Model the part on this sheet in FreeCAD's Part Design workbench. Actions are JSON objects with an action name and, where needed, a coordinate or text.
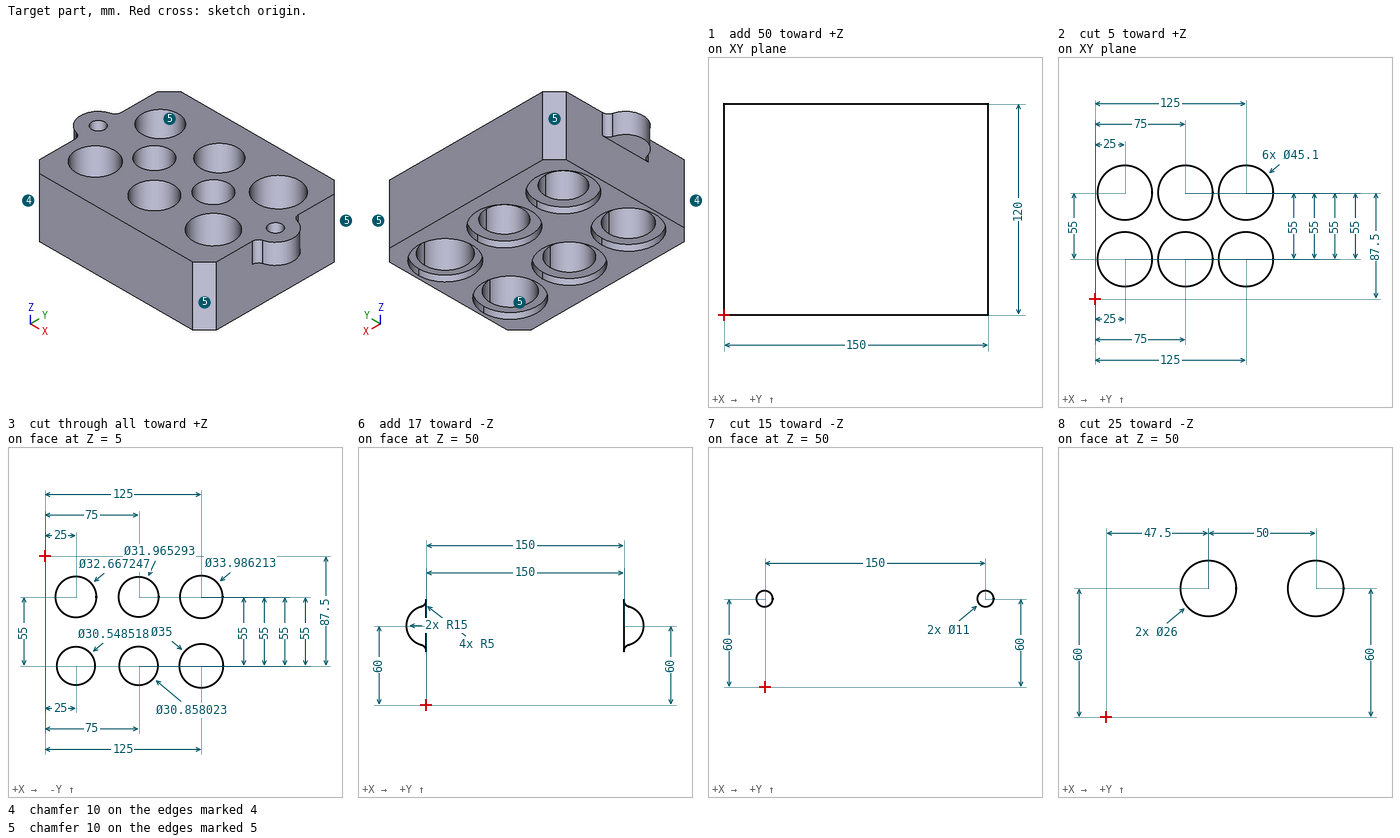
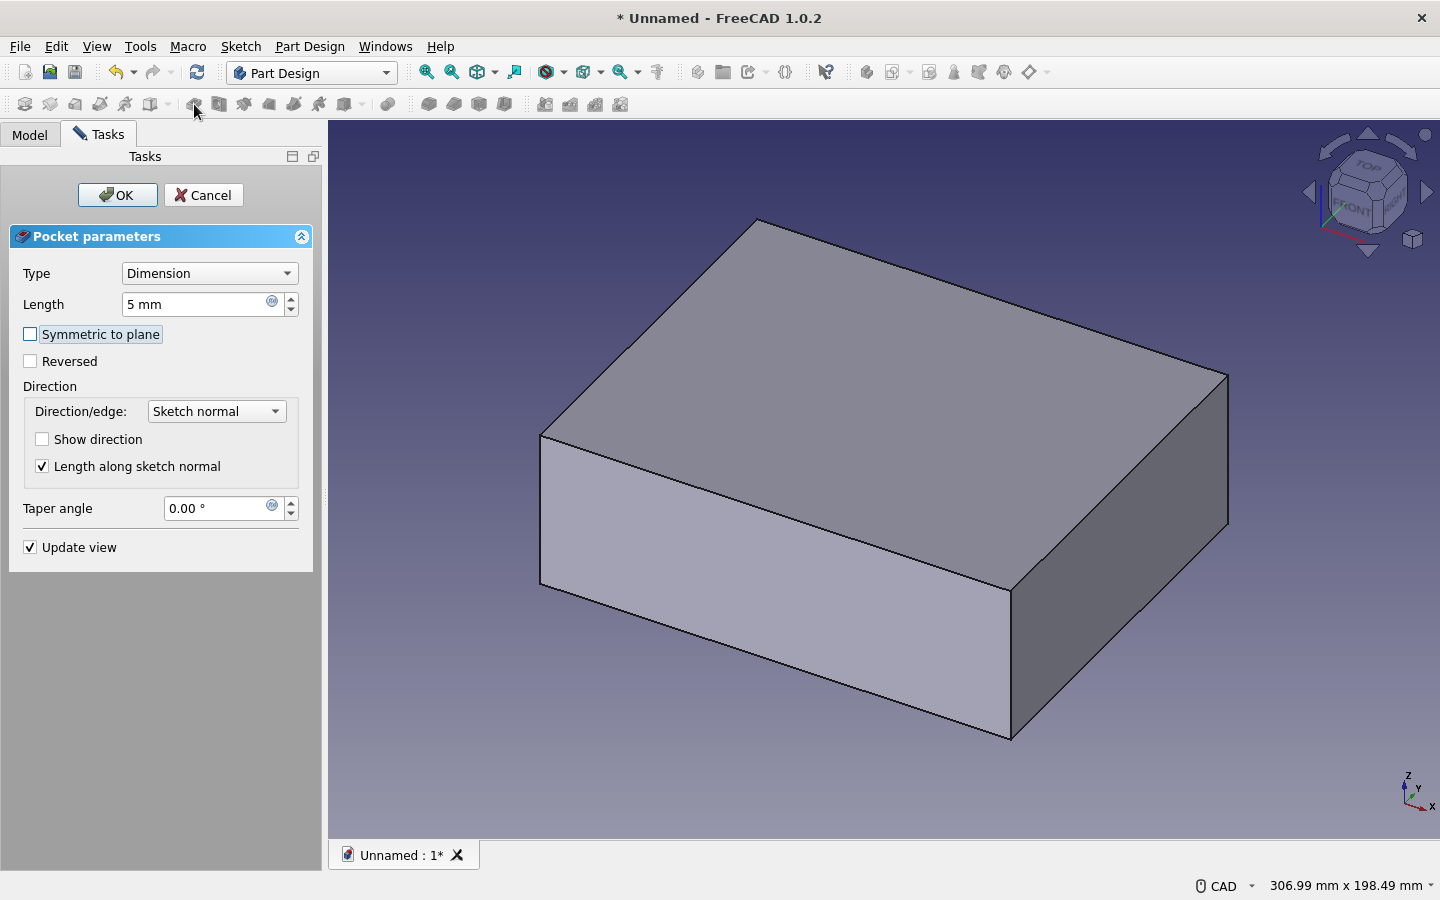
{"action": "left_click", "coordinate": [31, 361]}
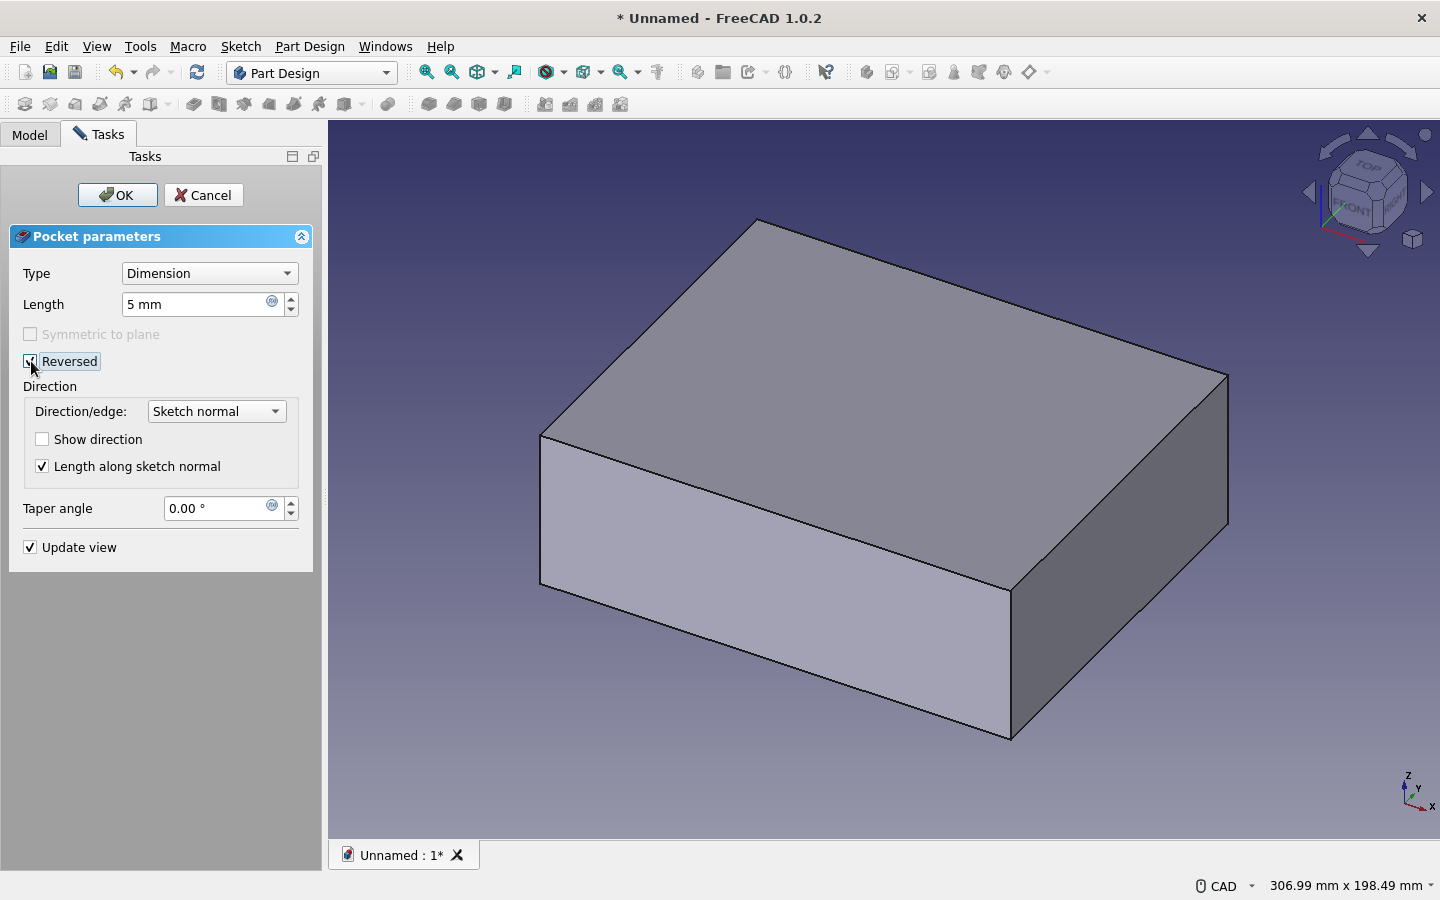
{"action": "left_click", "coordinate": [118, 195]}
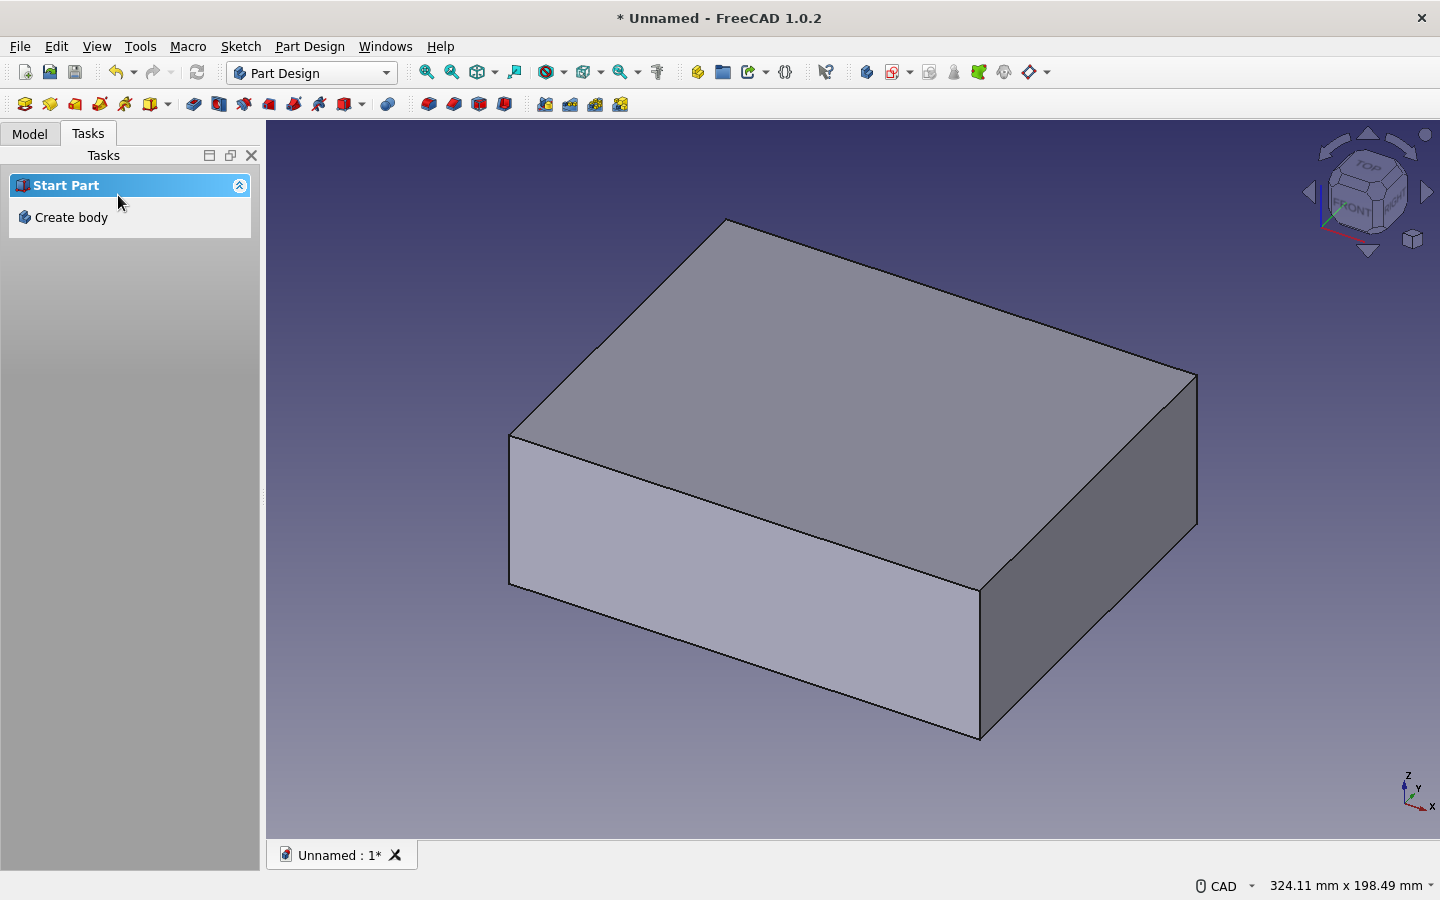
{"action": "key", "text": "5"}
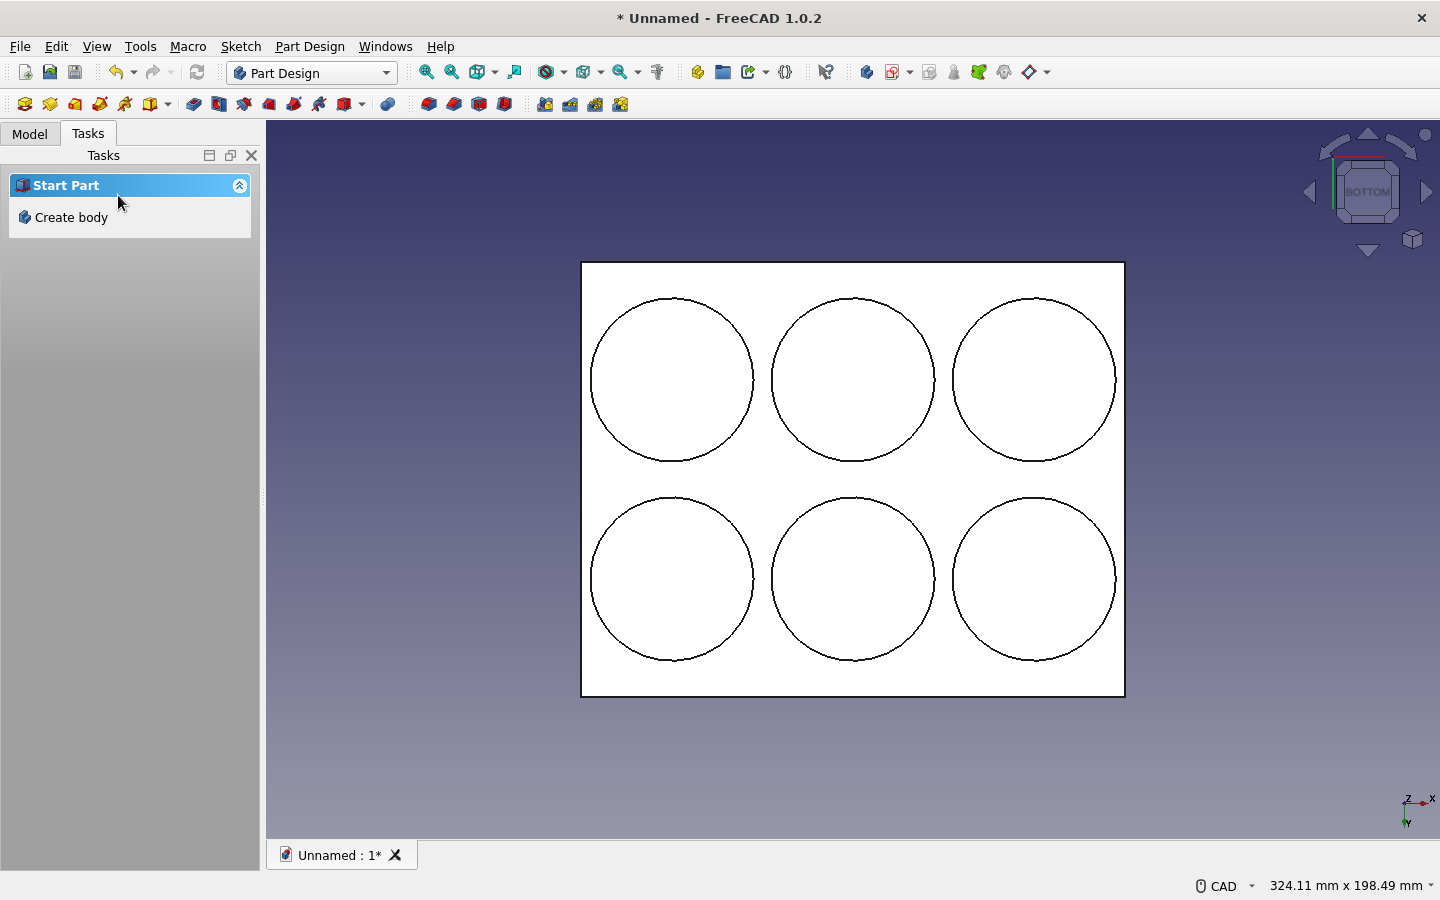
{"action": "left_click", "coordinate": [1034, 578]}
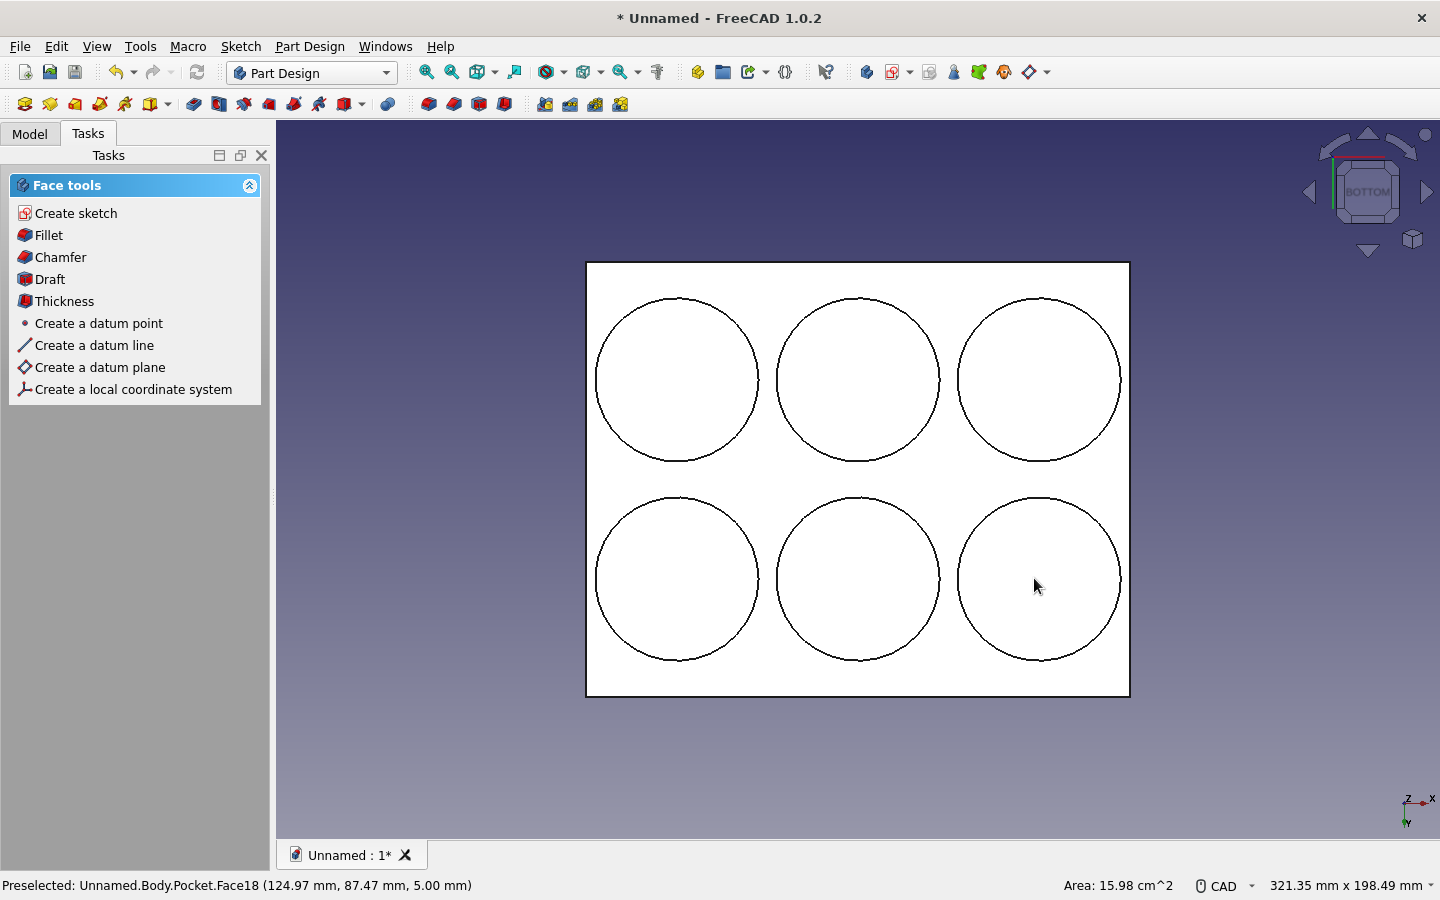
{"action": "left_click", "coordinate": [892, 72]}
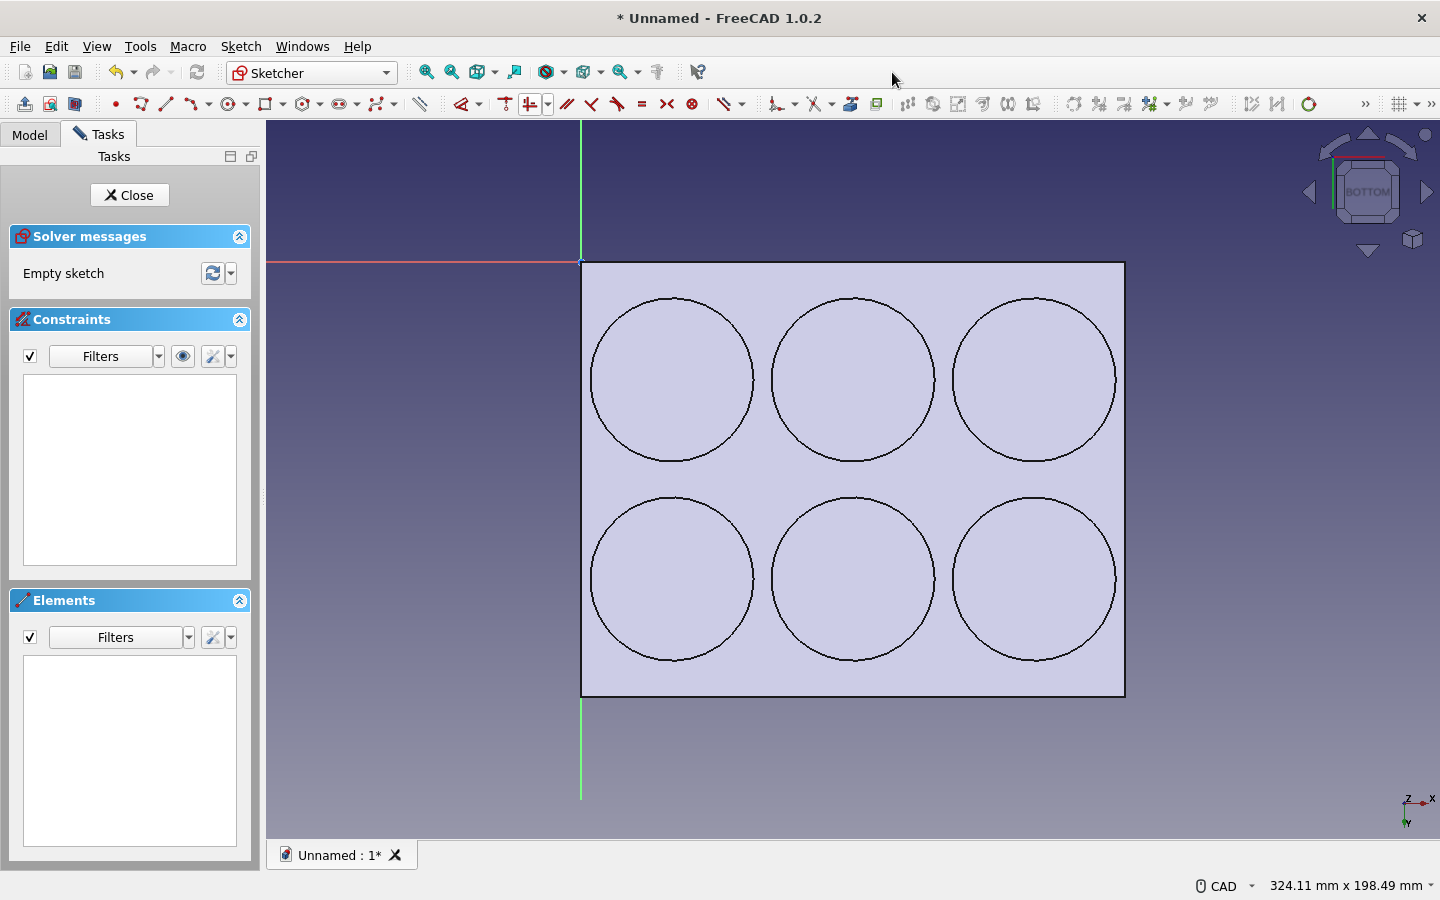
{"action": "left_click", "coordinate": [228, 104]}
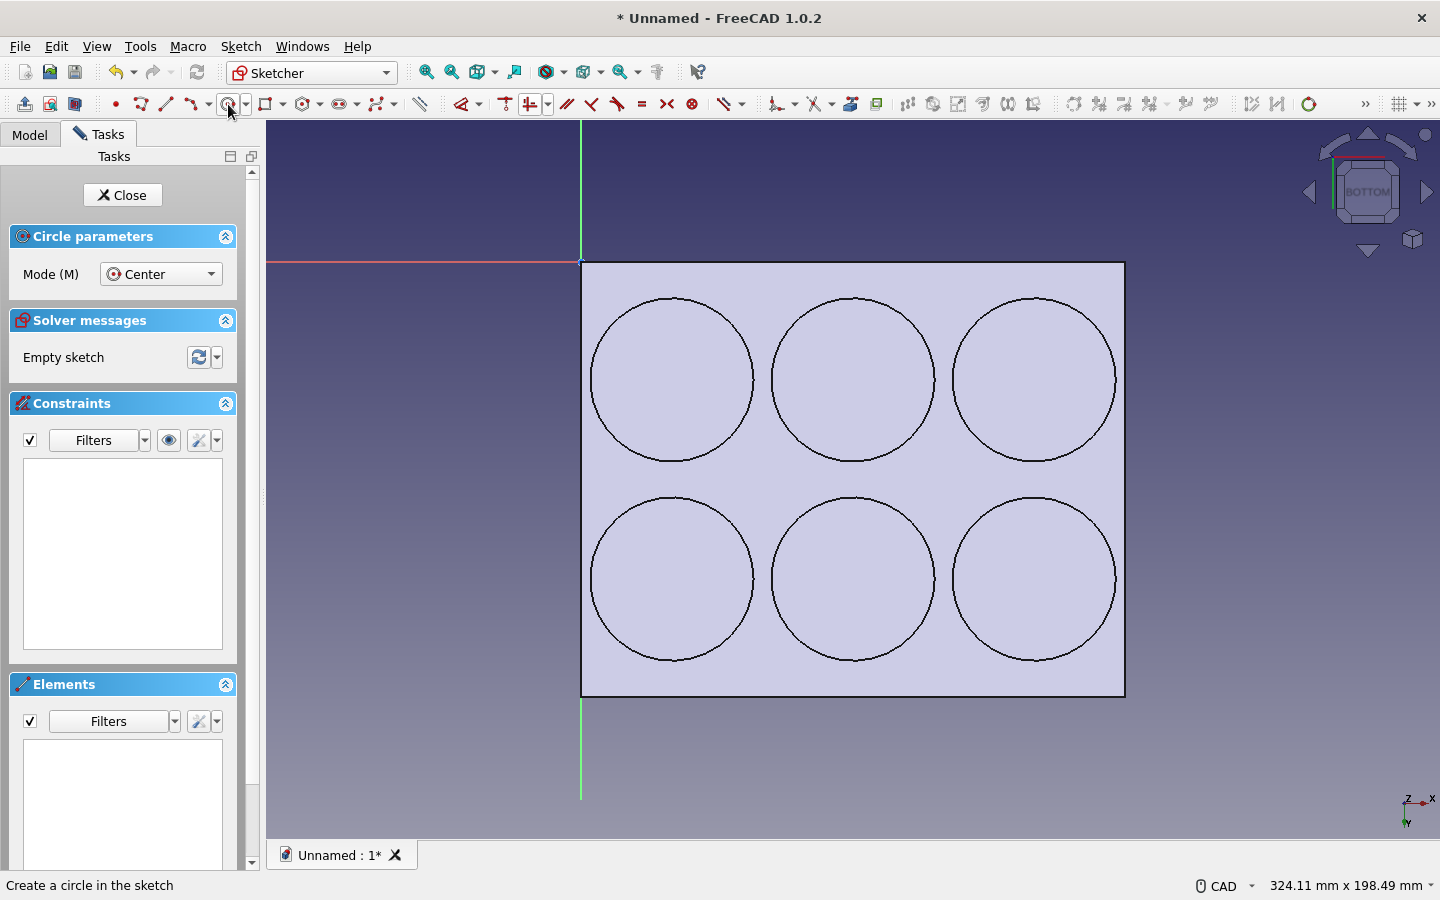
{"action": "left_click", "coordinate": [1034, 579]}
{"action": "left_click", "coordinate": [1079, 534]}